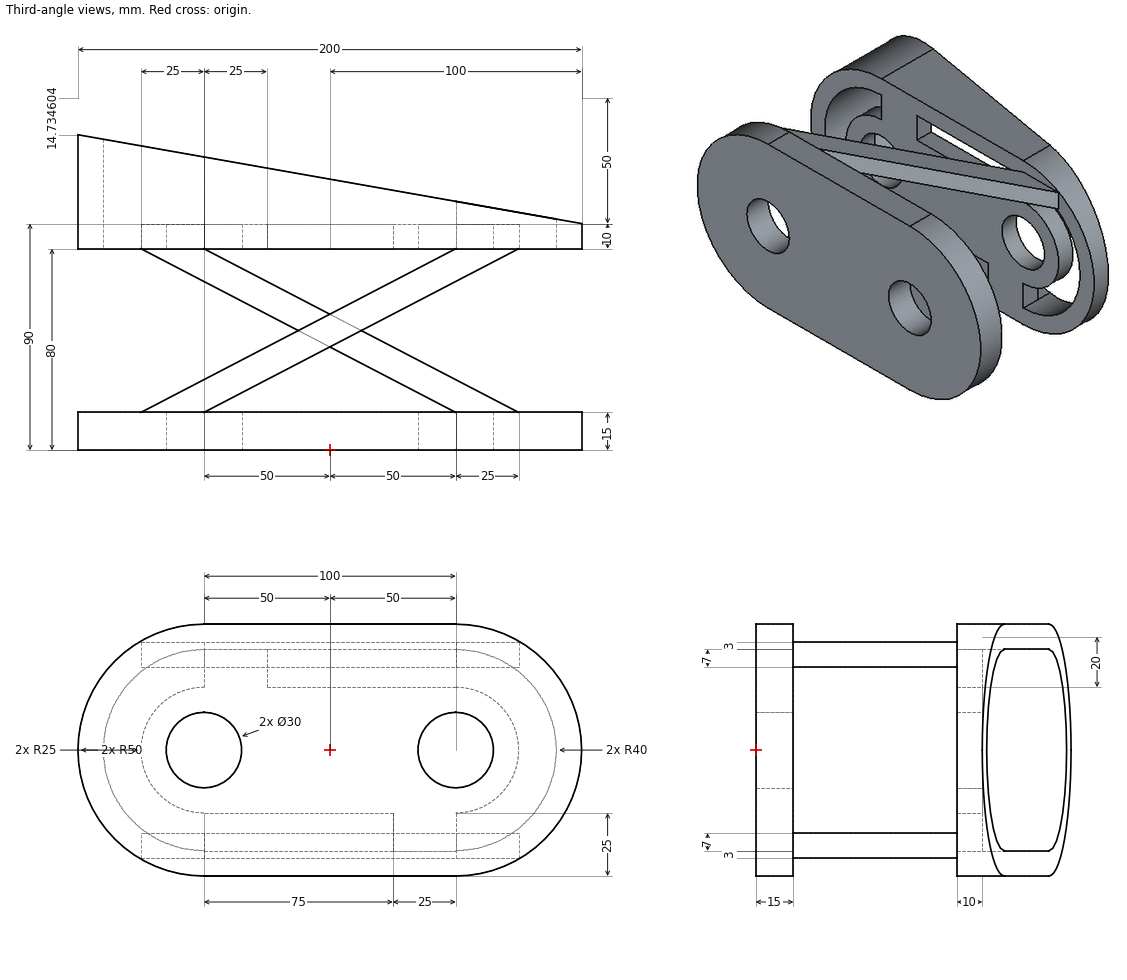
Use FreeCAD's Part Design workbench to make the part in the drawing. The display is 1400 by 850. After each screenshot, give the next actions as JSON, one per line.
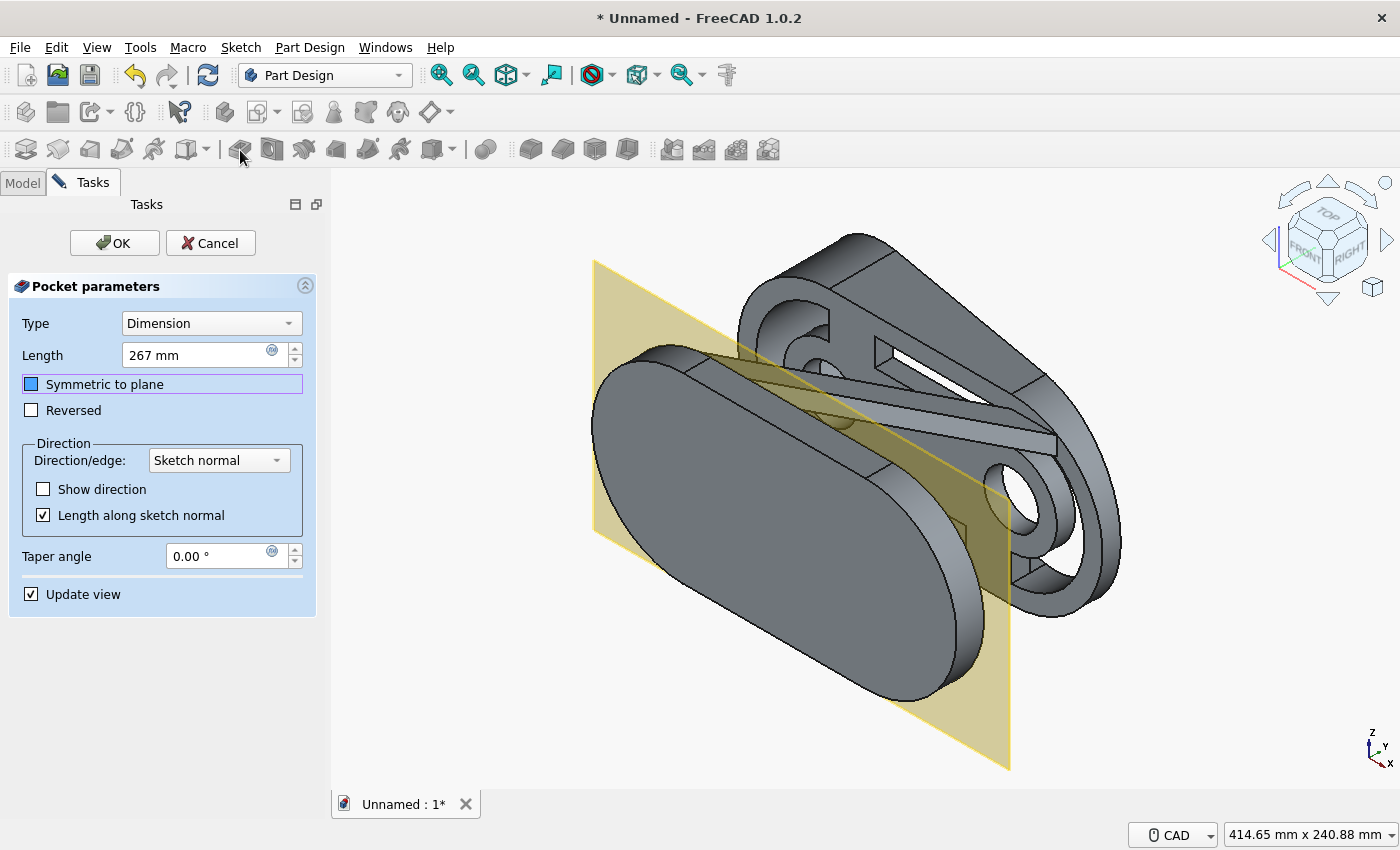
{"action": "left_click", "coordinate": [30, 384]}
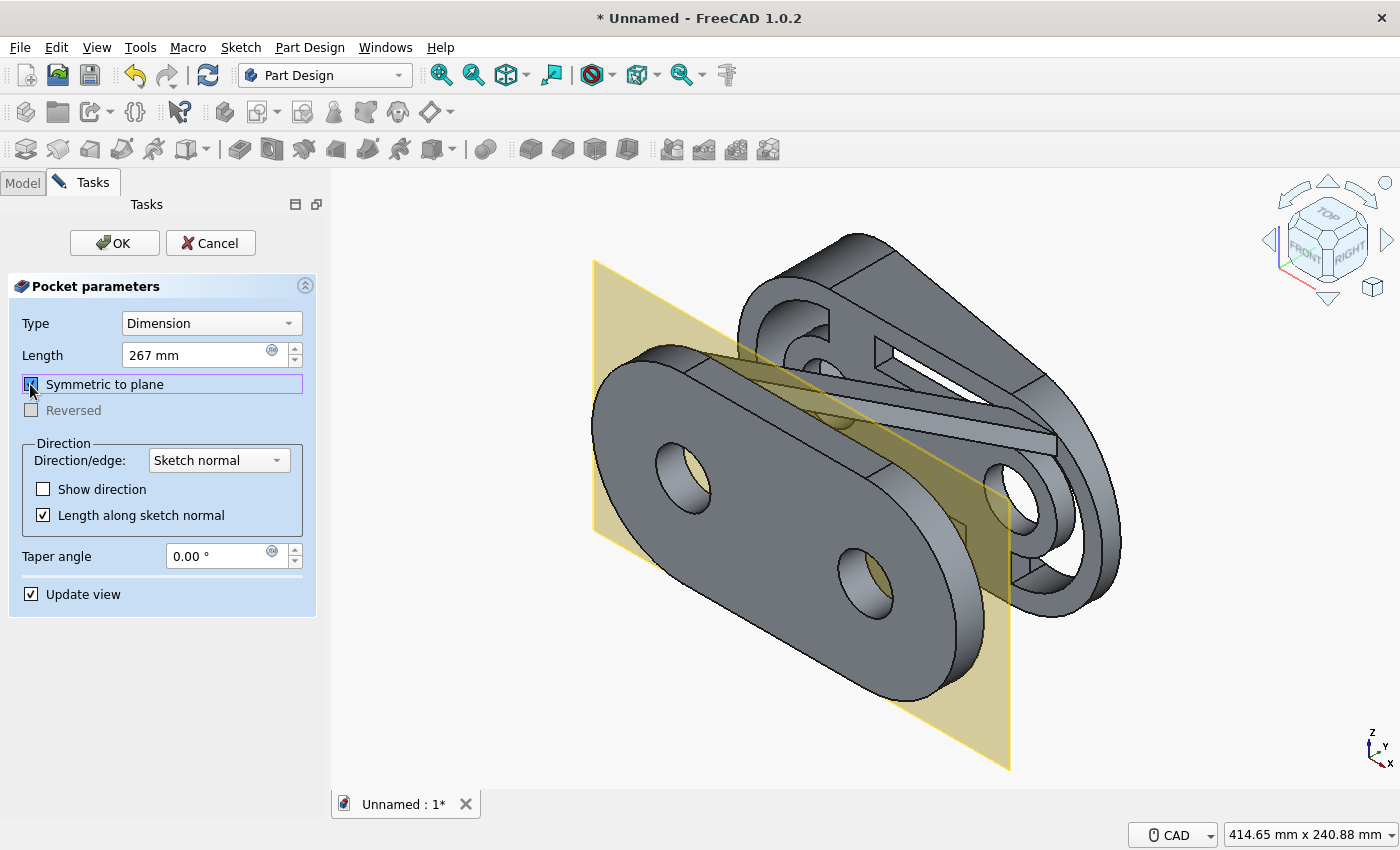
{"action": "left_click", "coordinate": [115, 243]}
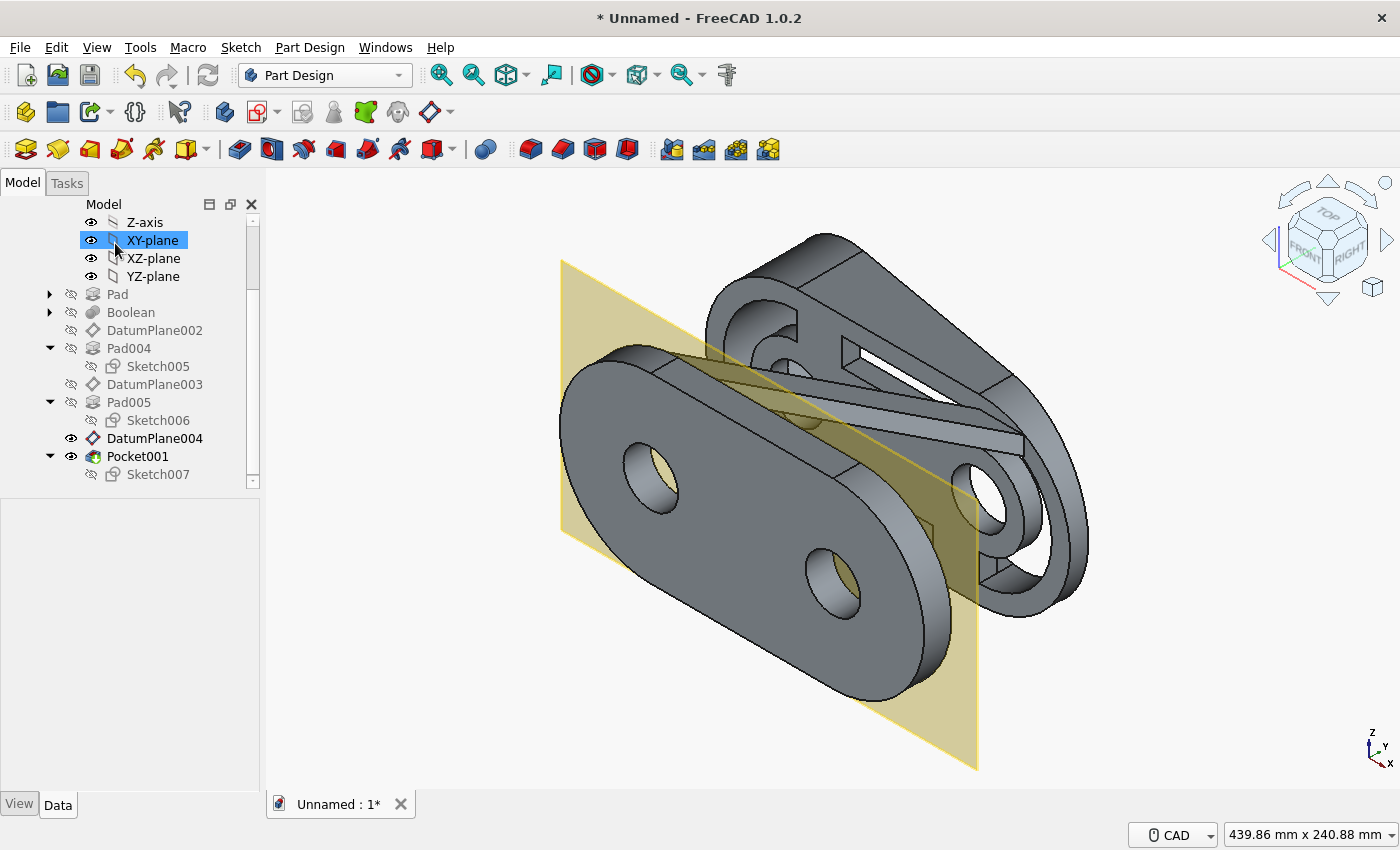
{"action": "left_click", "coordinate": [116, 438]}
{"action": "key", "text": "space"}